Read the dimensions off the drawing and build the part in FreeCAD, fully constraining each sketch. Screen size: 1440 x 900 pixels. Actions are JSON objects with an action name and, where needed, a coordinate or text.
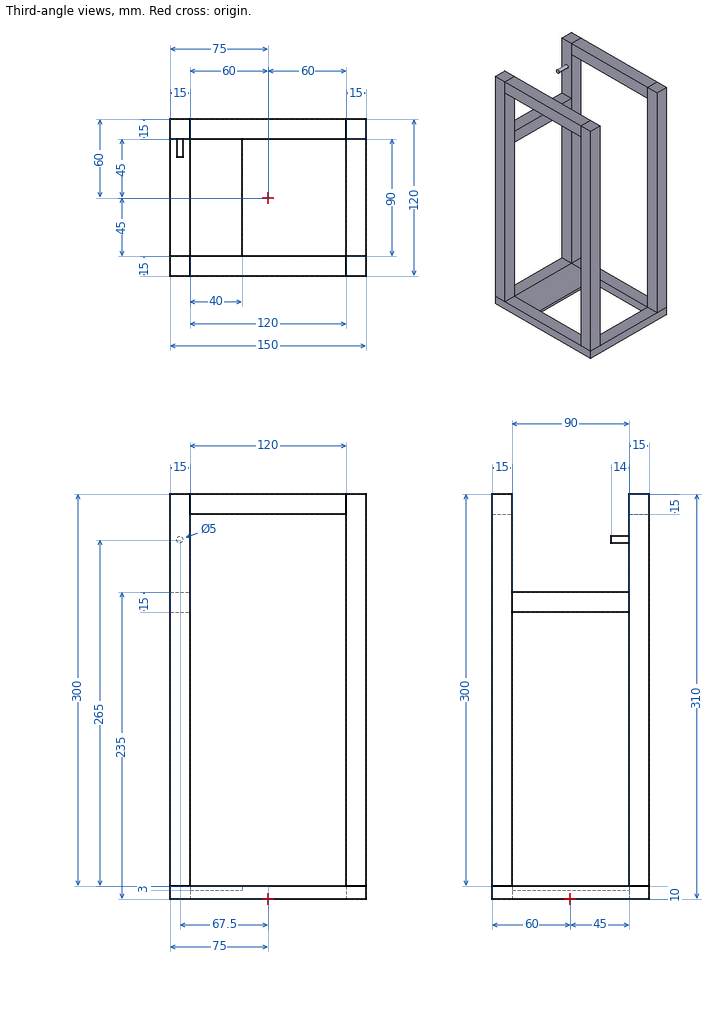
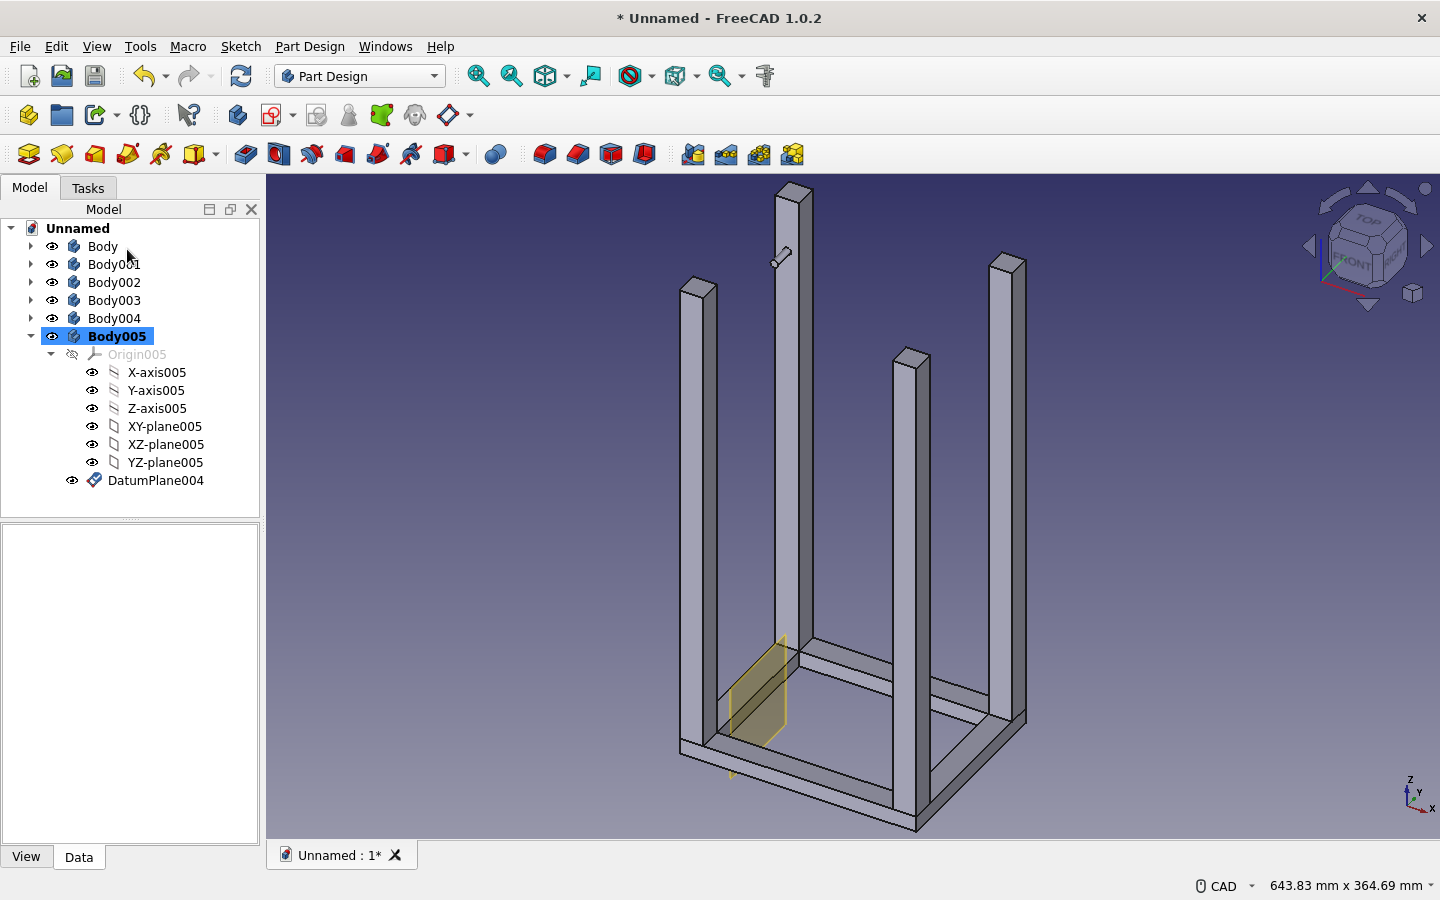
{"action": "left_click", "coordinate": [117, 480]}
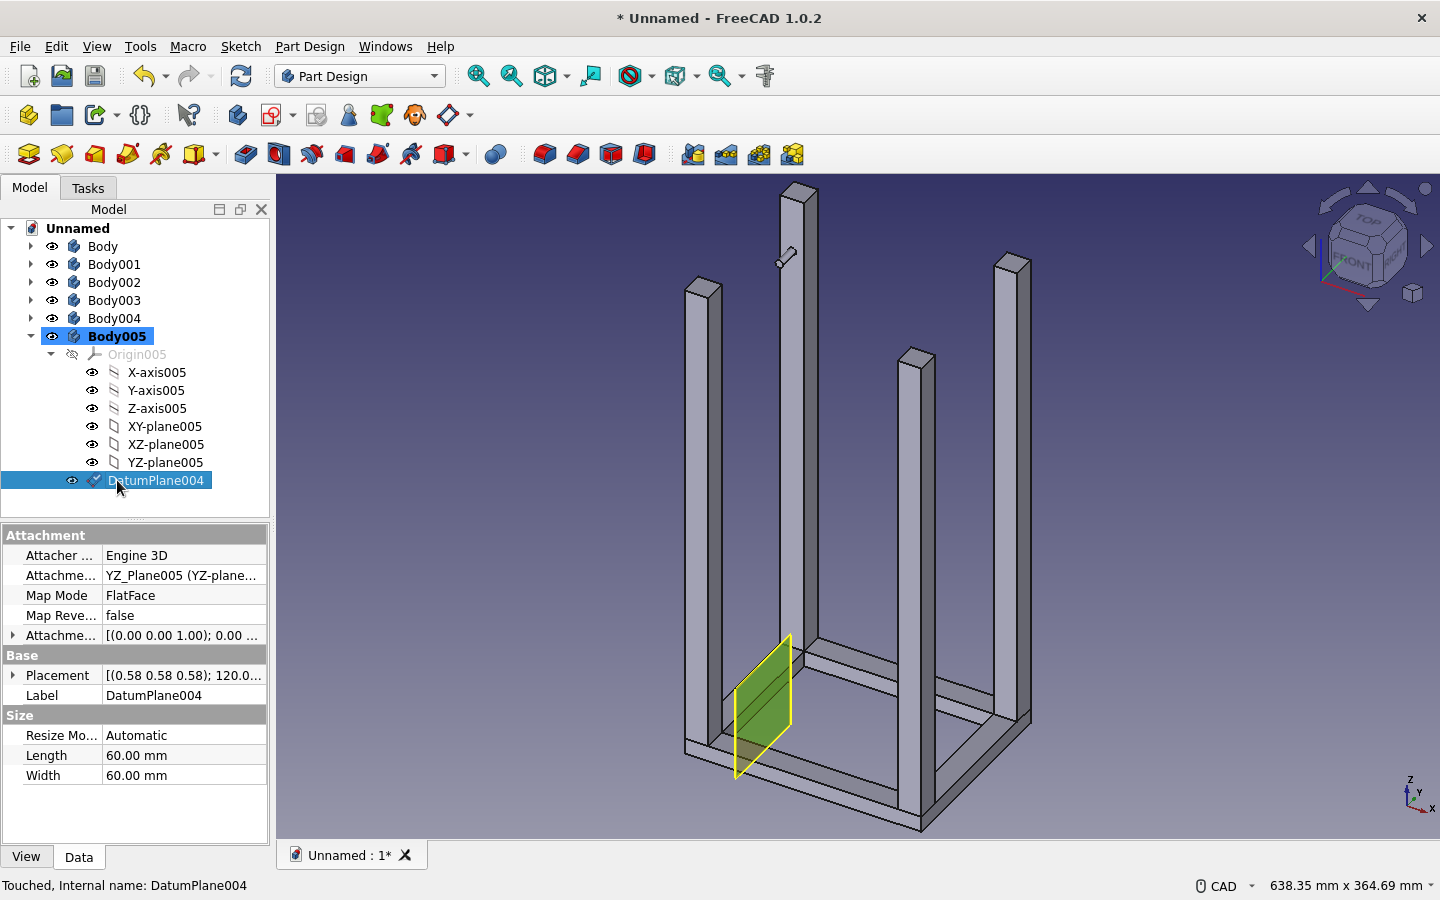
{"action": "left_click", "coordinate": [270, 116]}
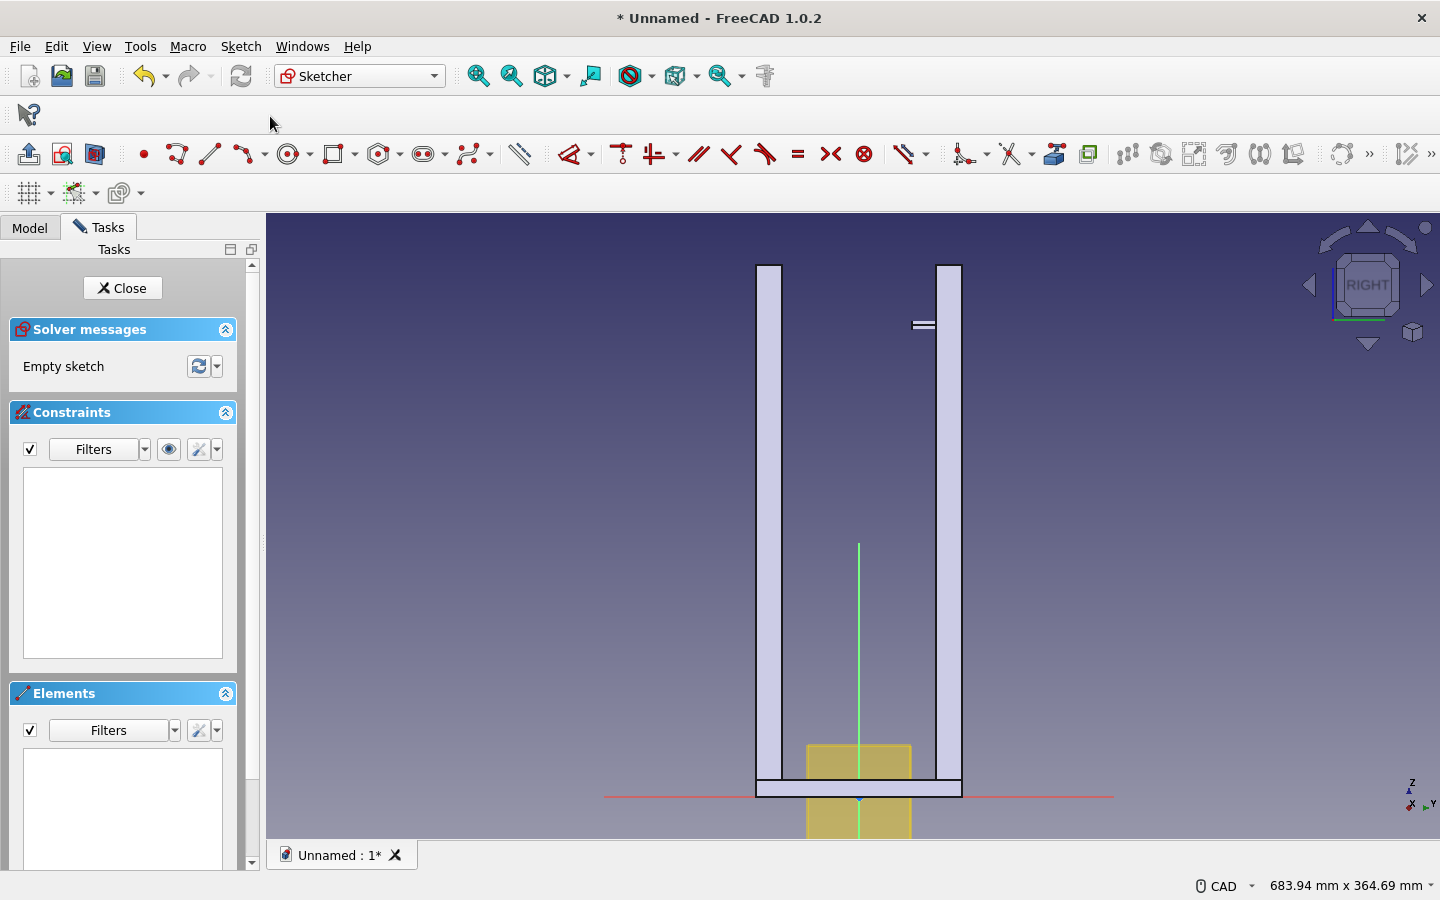
{"action": "scroll", "coordinate": [960, 262], "scroll_direction": "up", "scroll_amount": 14}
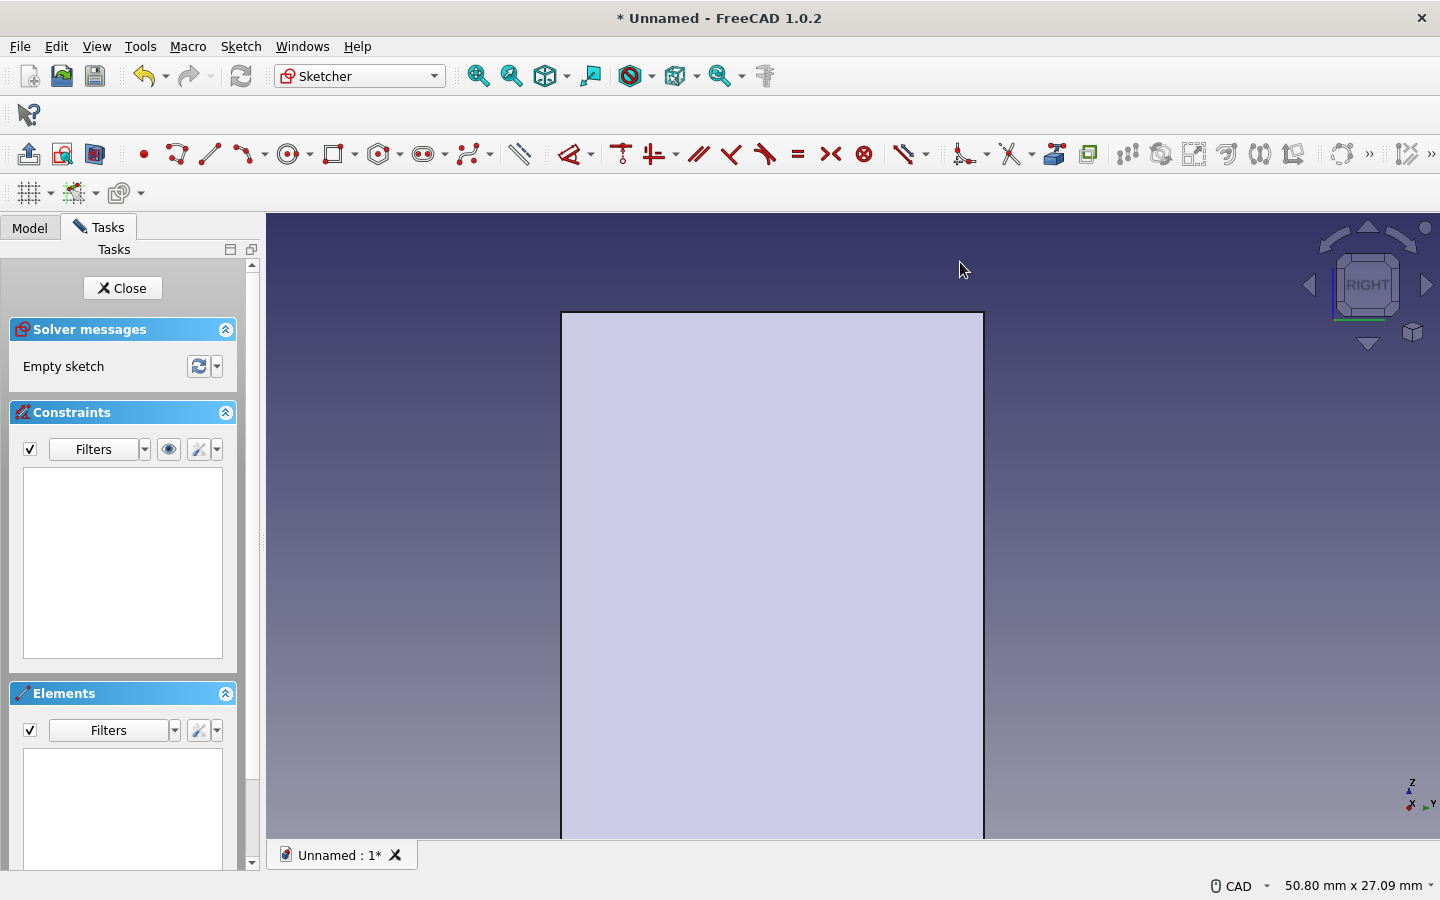
{"action": "left_click", "coordinate": [332, 154]}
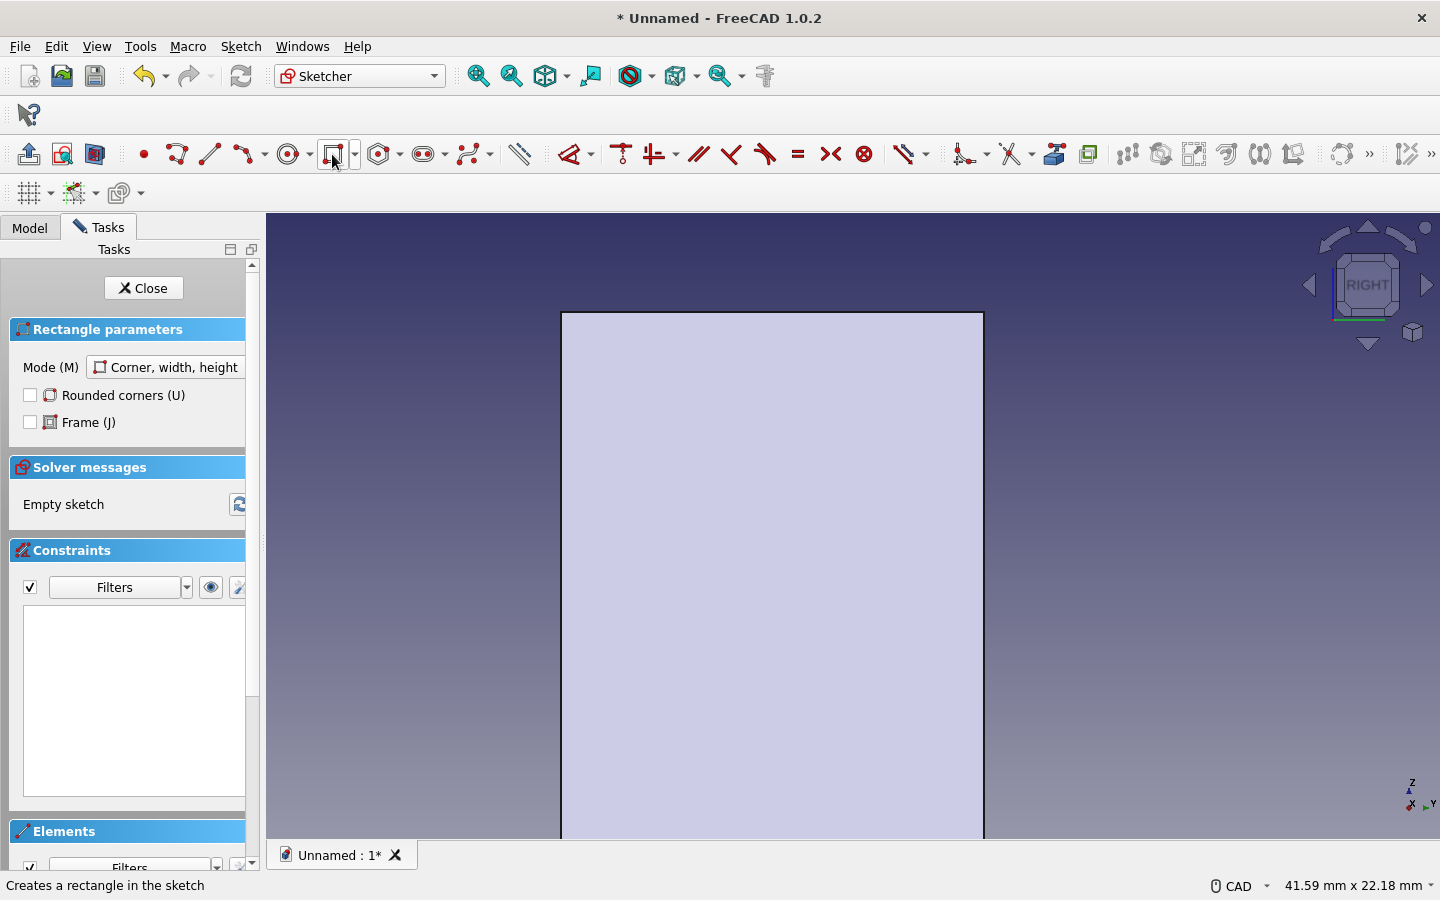
{"action": "left_click", "coordinate": [561, 312]}
{"action": "left_click", "coordinate": [984, 735]}
{"action": "key", "text": "Escape"}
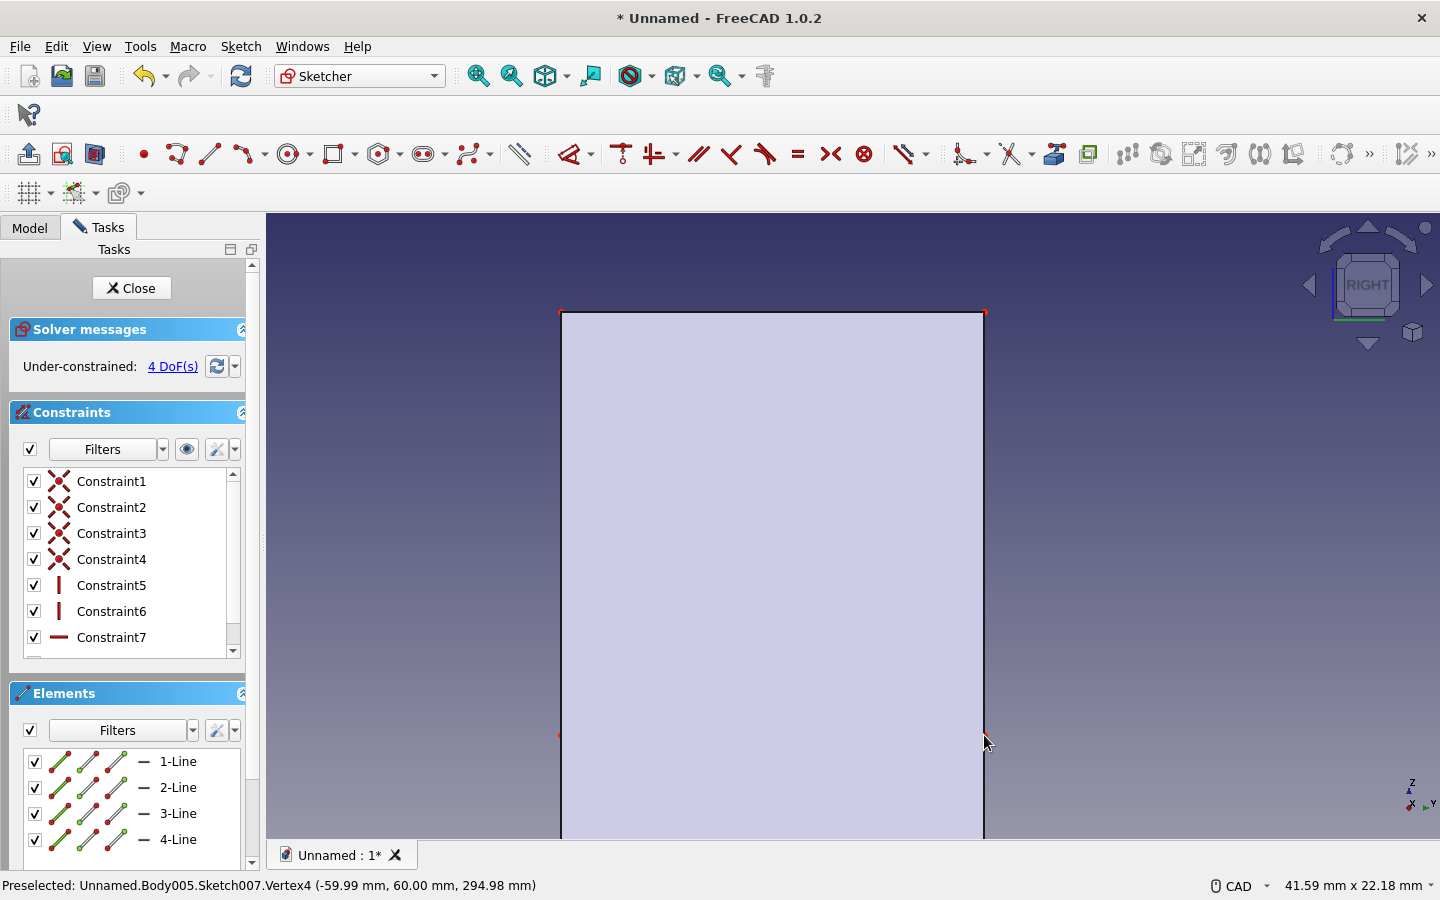
{"action": "left_click", "coordinate": [568, 154]}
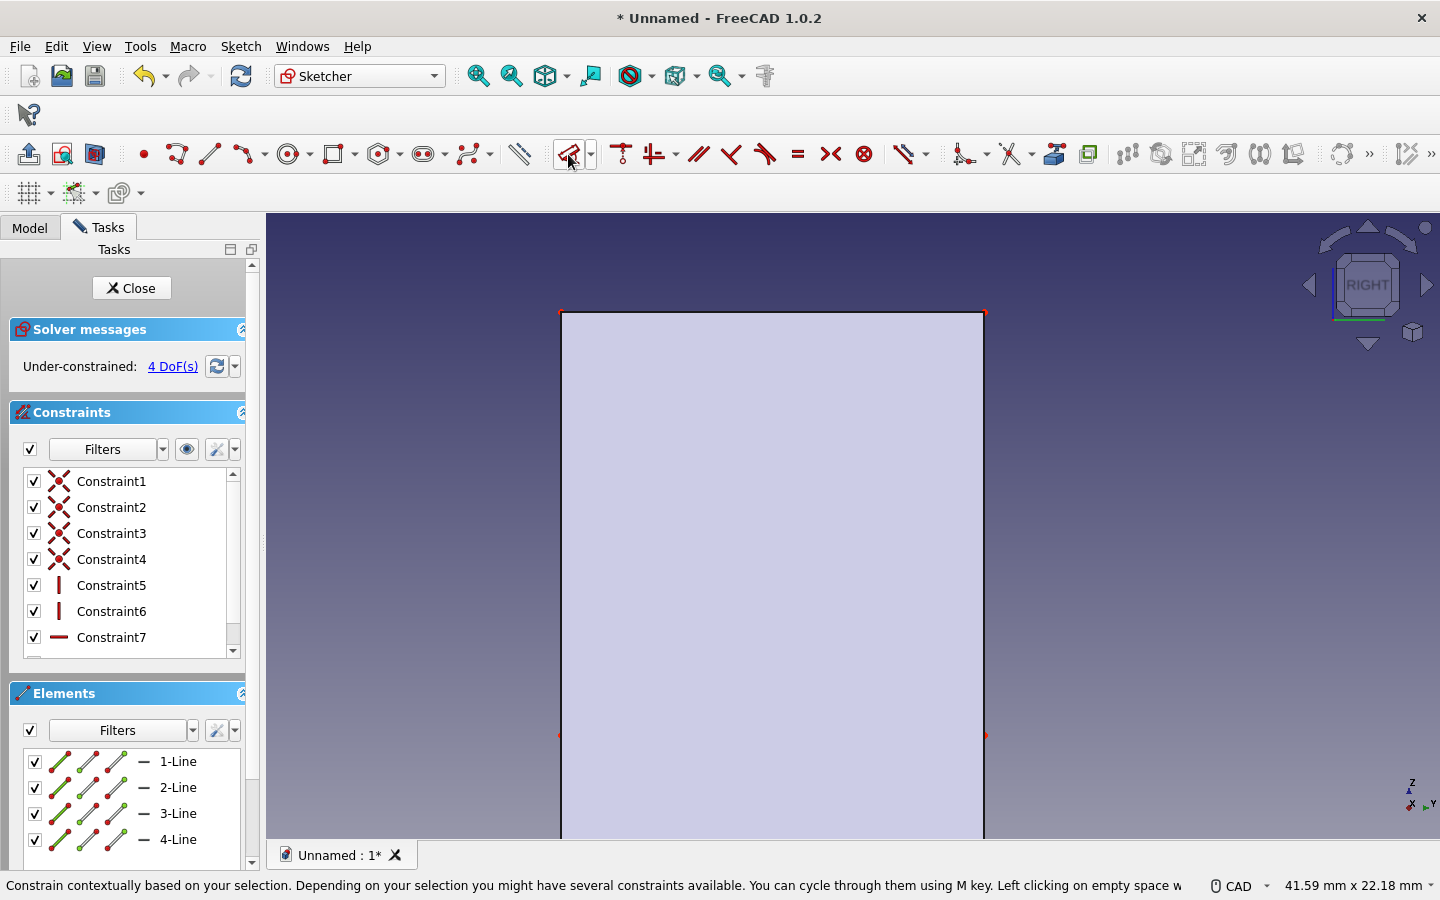
{"action": "left_click", "coordinate": [561, 440]}
{"action": "left_click", "coordinate": [527, 524]}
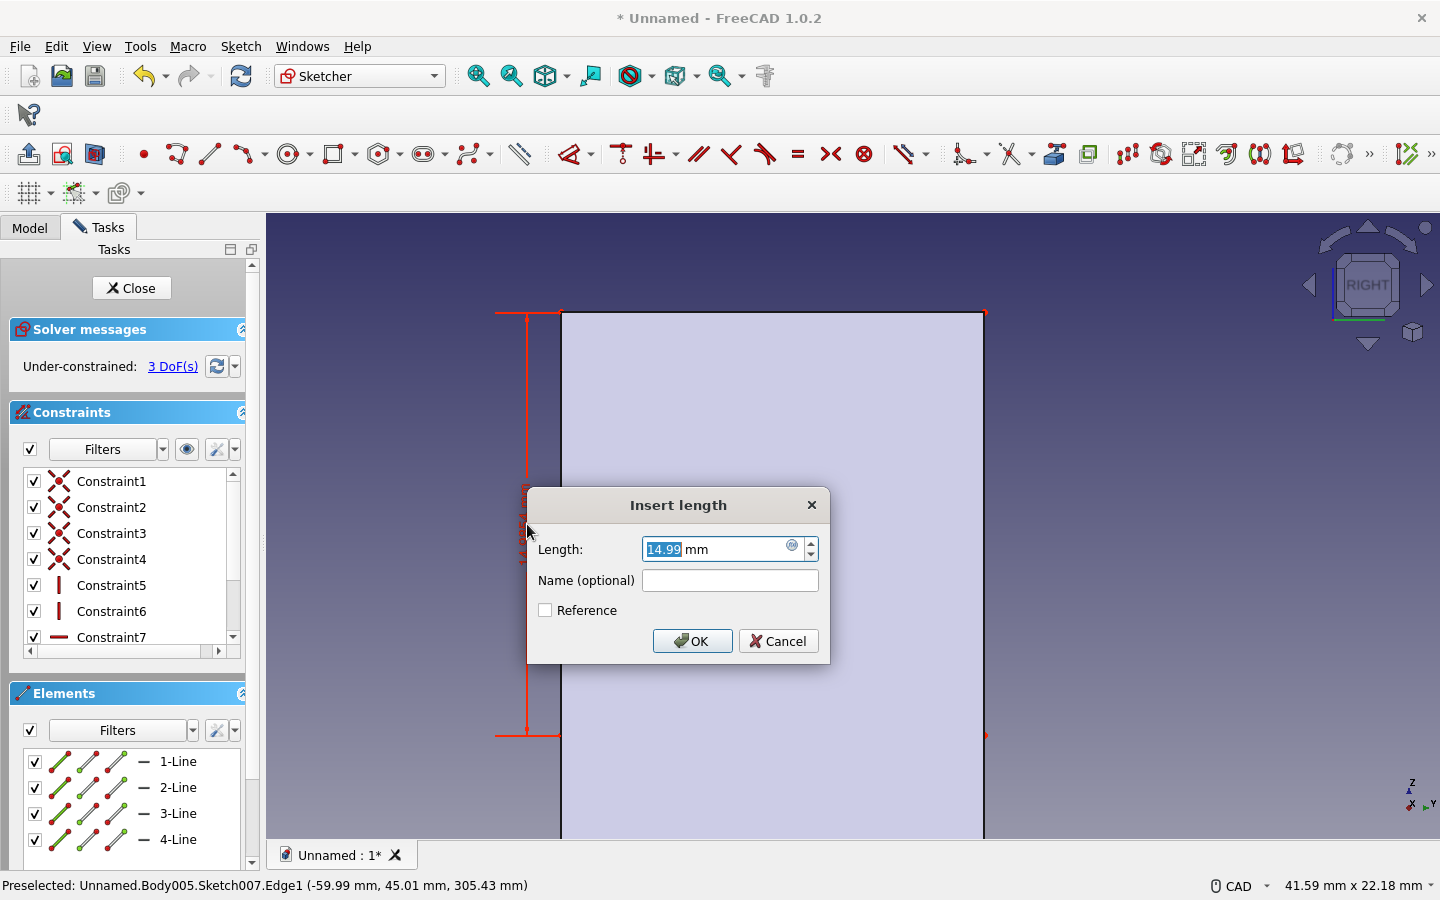
{"action": "type", "text": "15"}
{"action": "key", "text": "Return"}